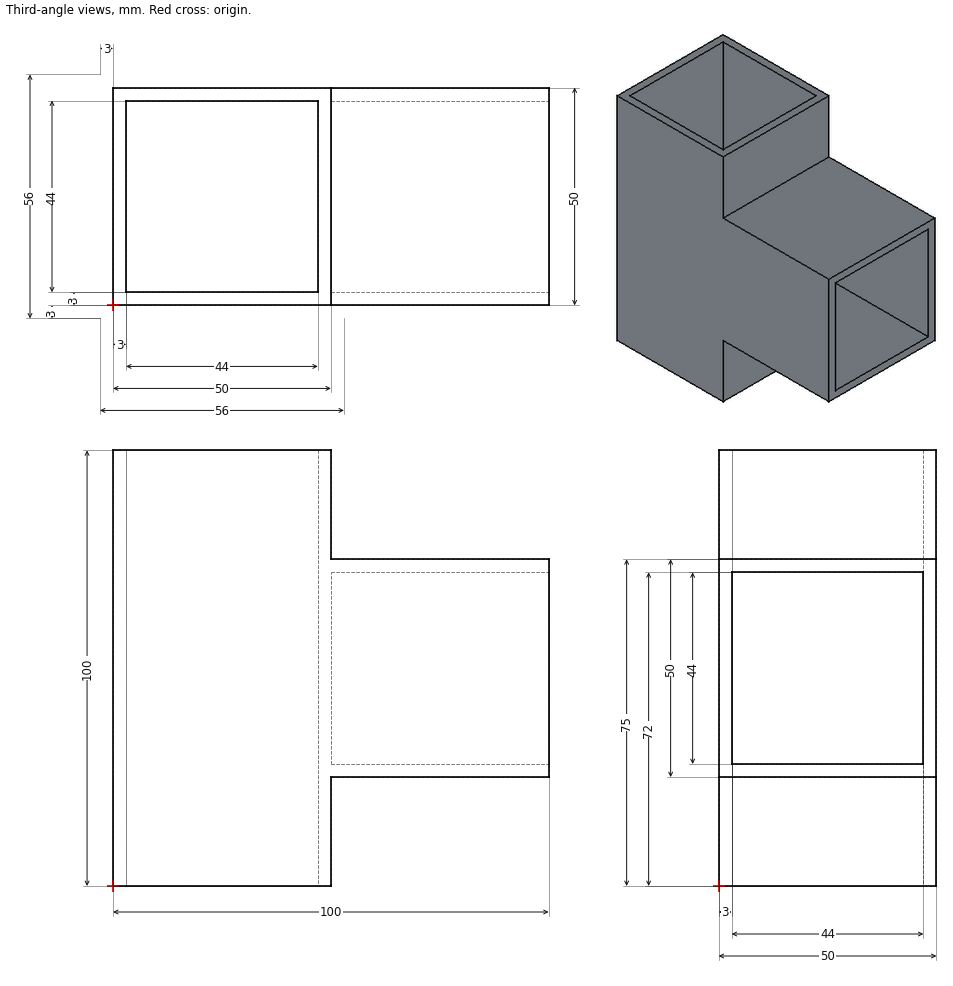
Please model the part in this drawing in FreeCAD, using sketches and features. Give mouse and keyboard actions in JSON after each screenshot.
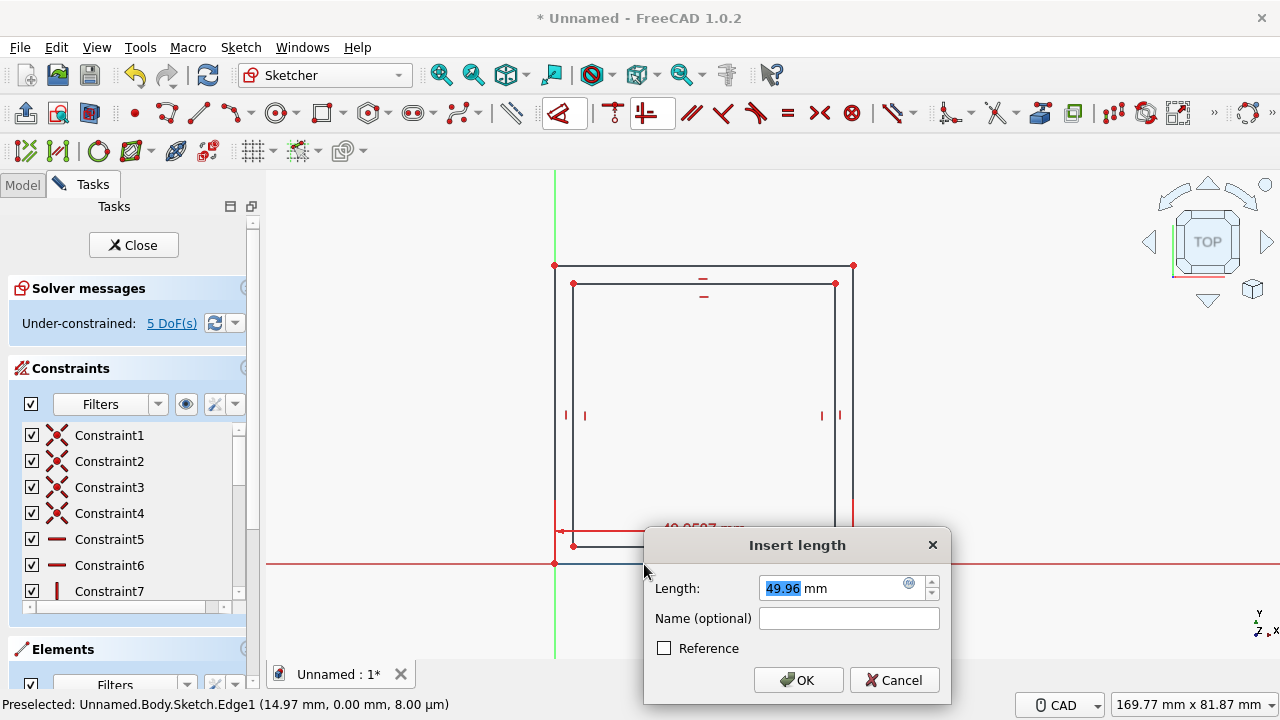
{"action": "type", "text": "50"}
{"action": "key", "text": "Return"}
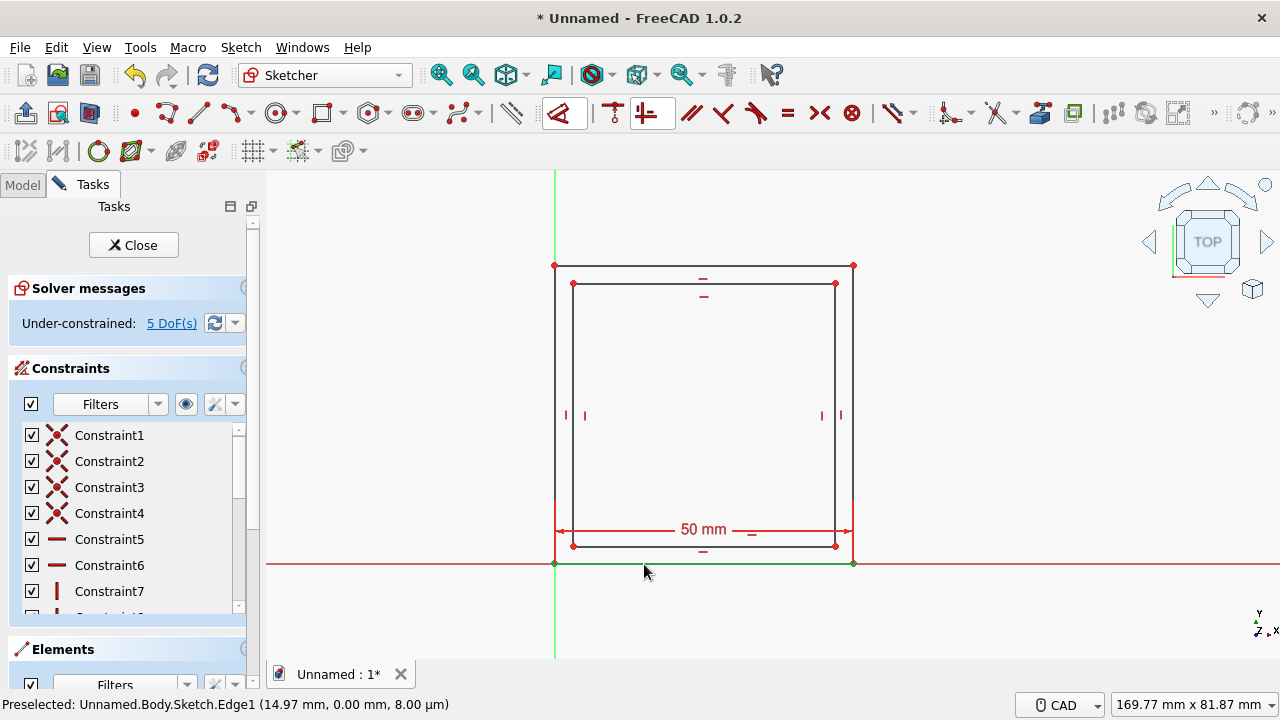
{"action": "left_click", "coordinate": [853, 475]}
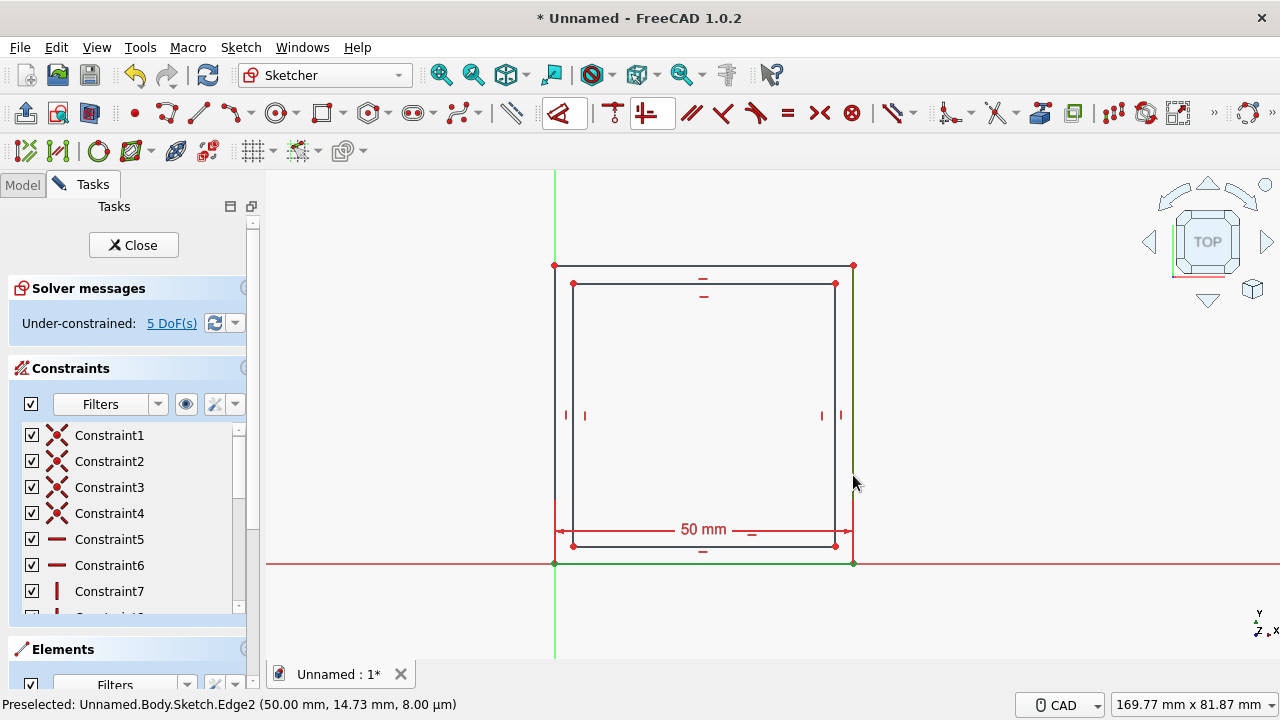
{"action": "key", "text": "i"}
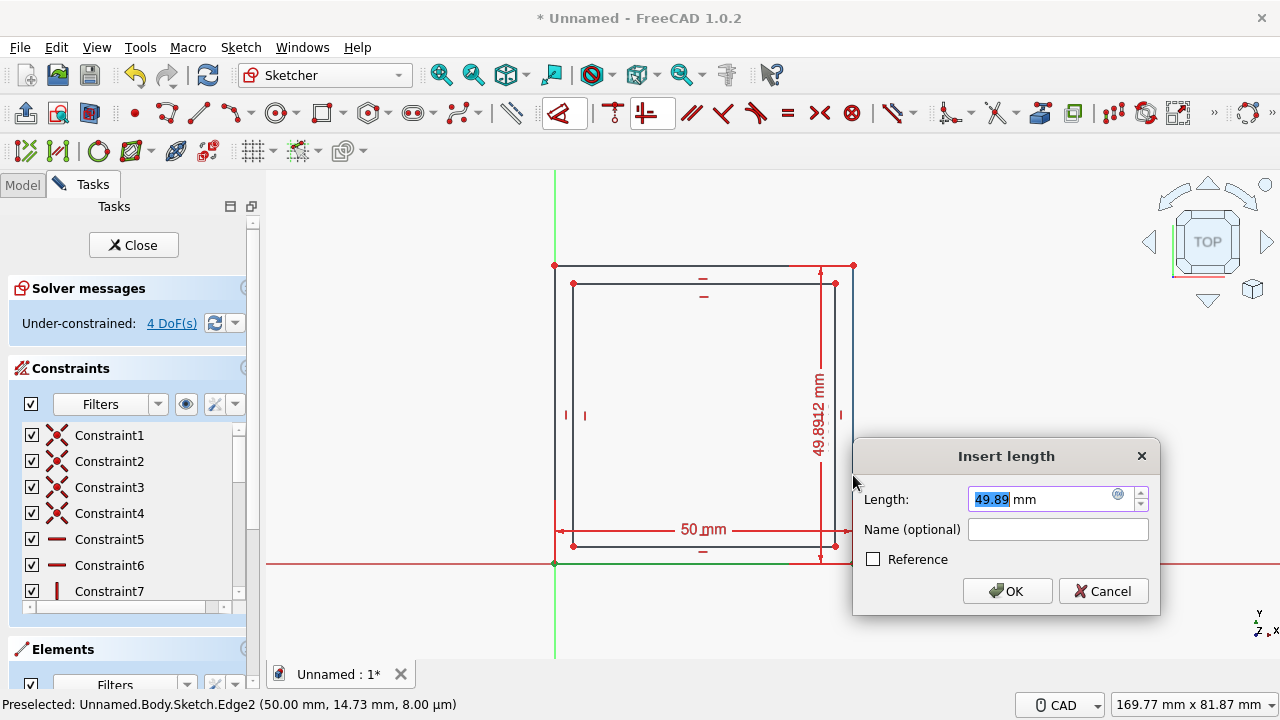
{"action": "type", "text": "50"}
{"action": "key", "text": "Return"}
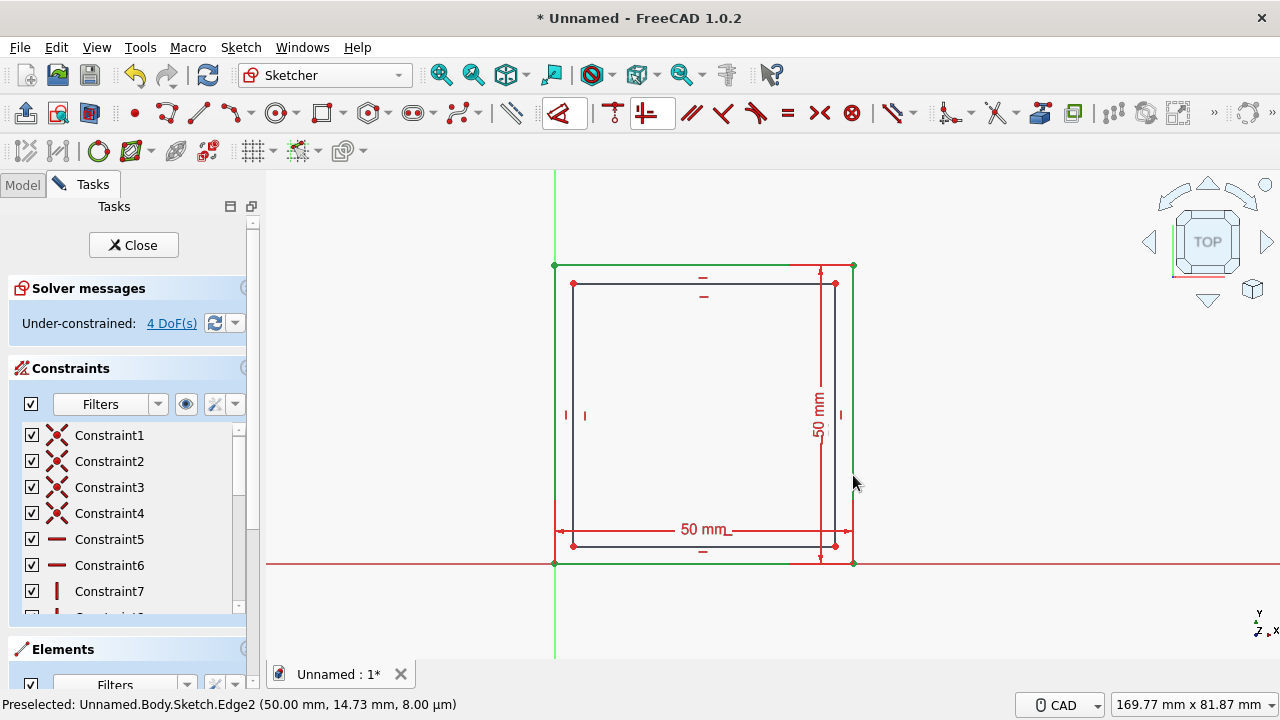
{"action": "left_click", "coordinate": [573, 363]}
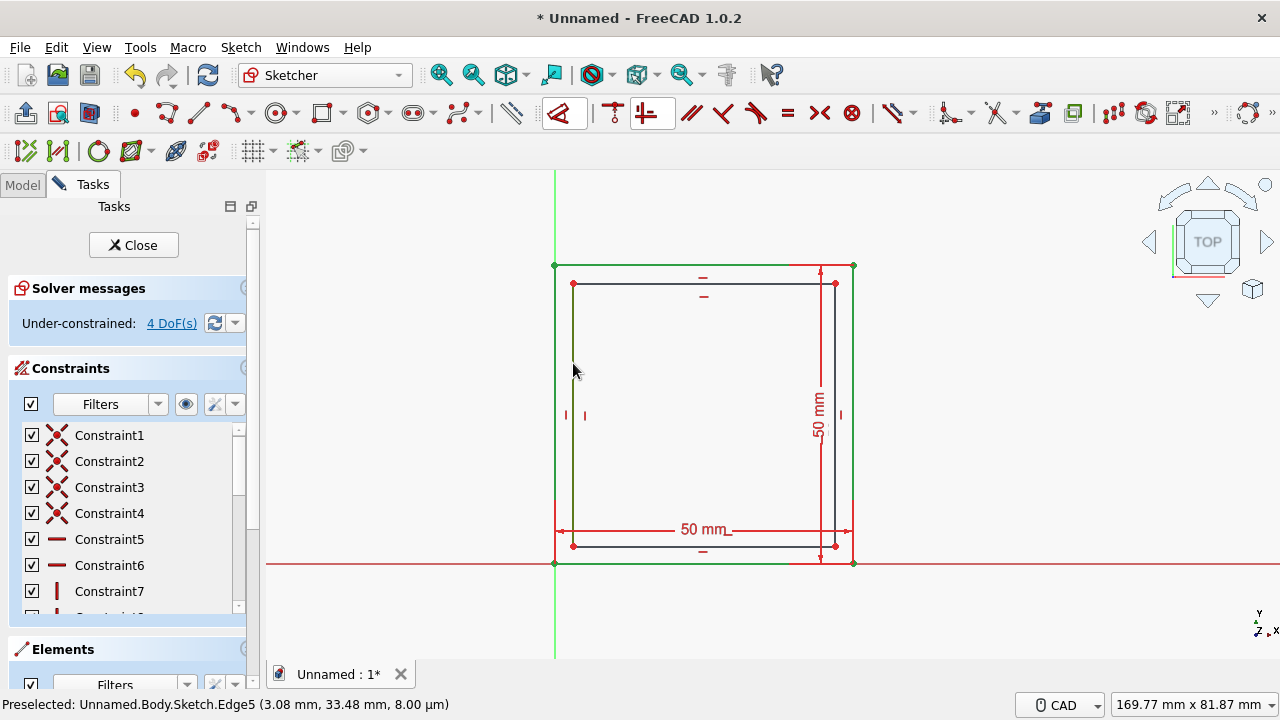
{"action": "key", "text": "i"}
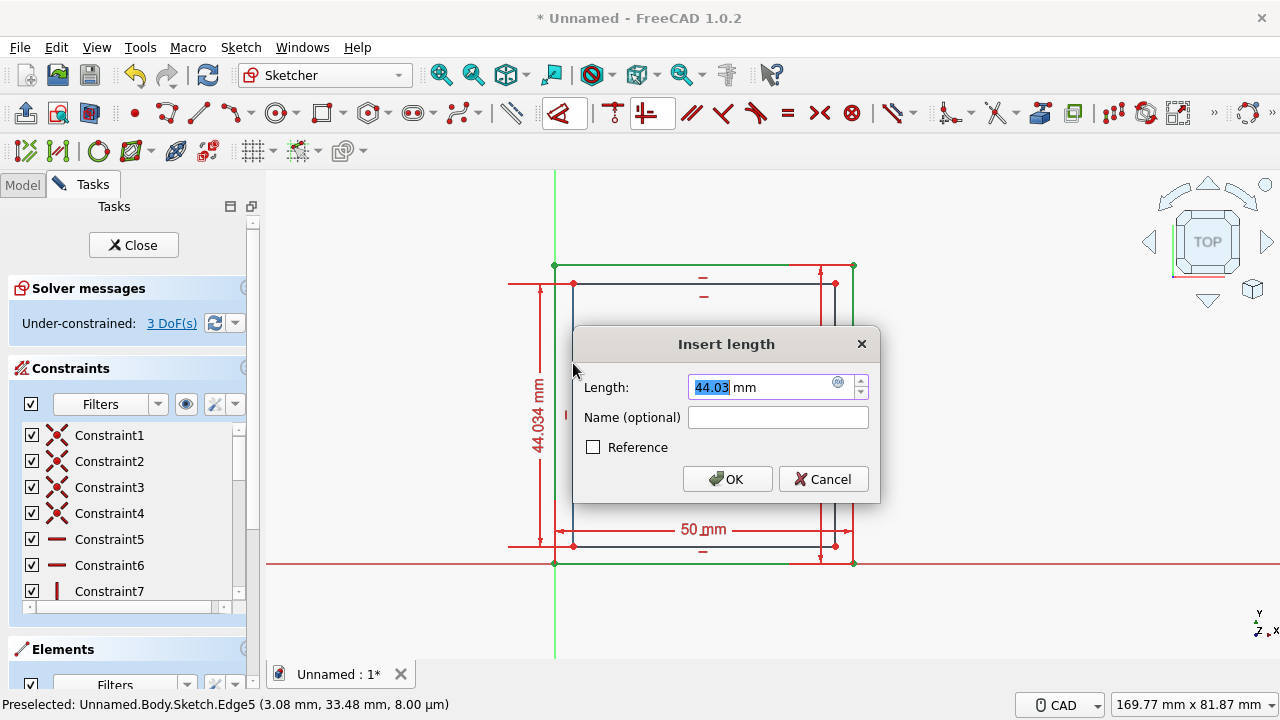
{"action": "type", "text": "44"}
{"action": "key", "text": "Return"}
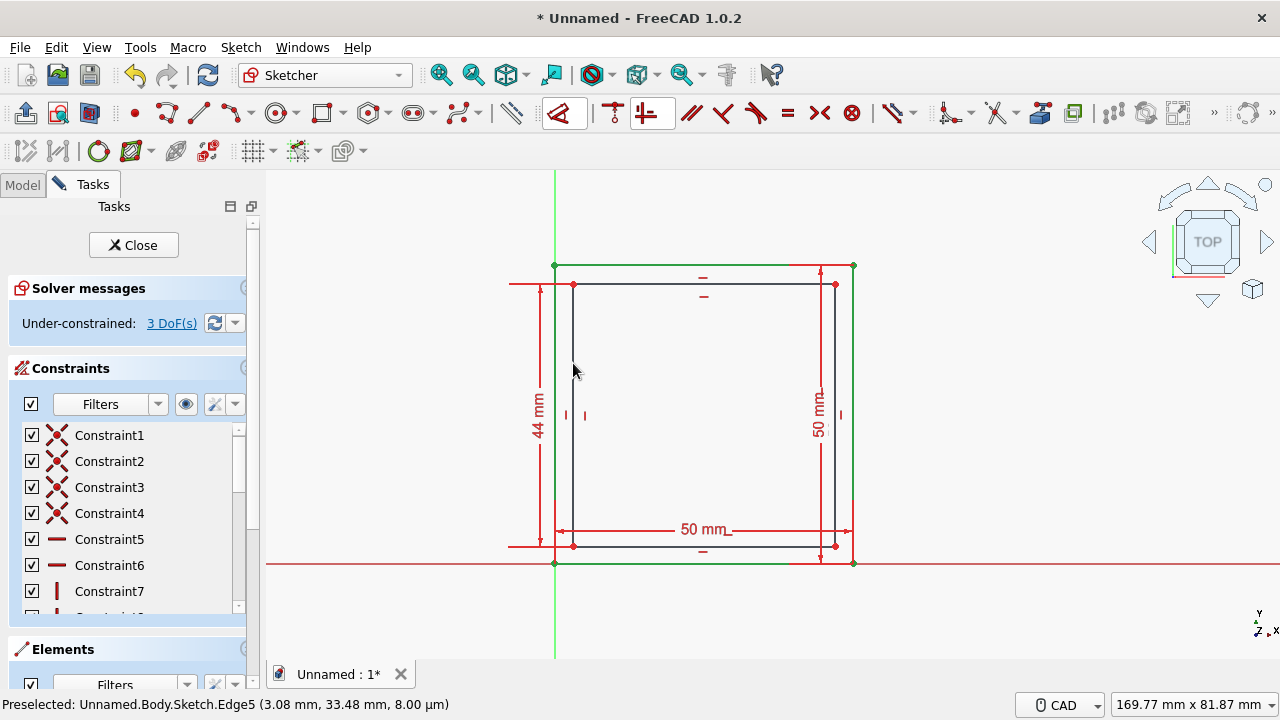
{"action": "left_click", "coordinate": [652, 547]}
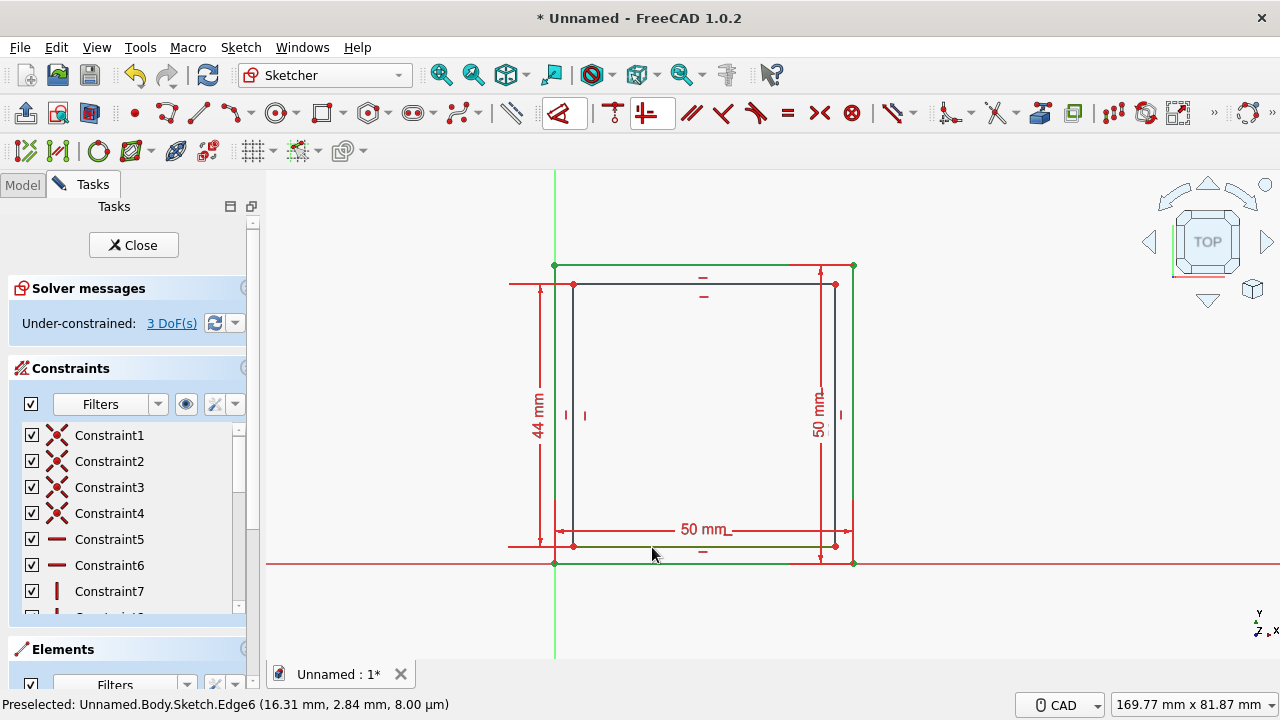
{"action": "key", "text": "l"}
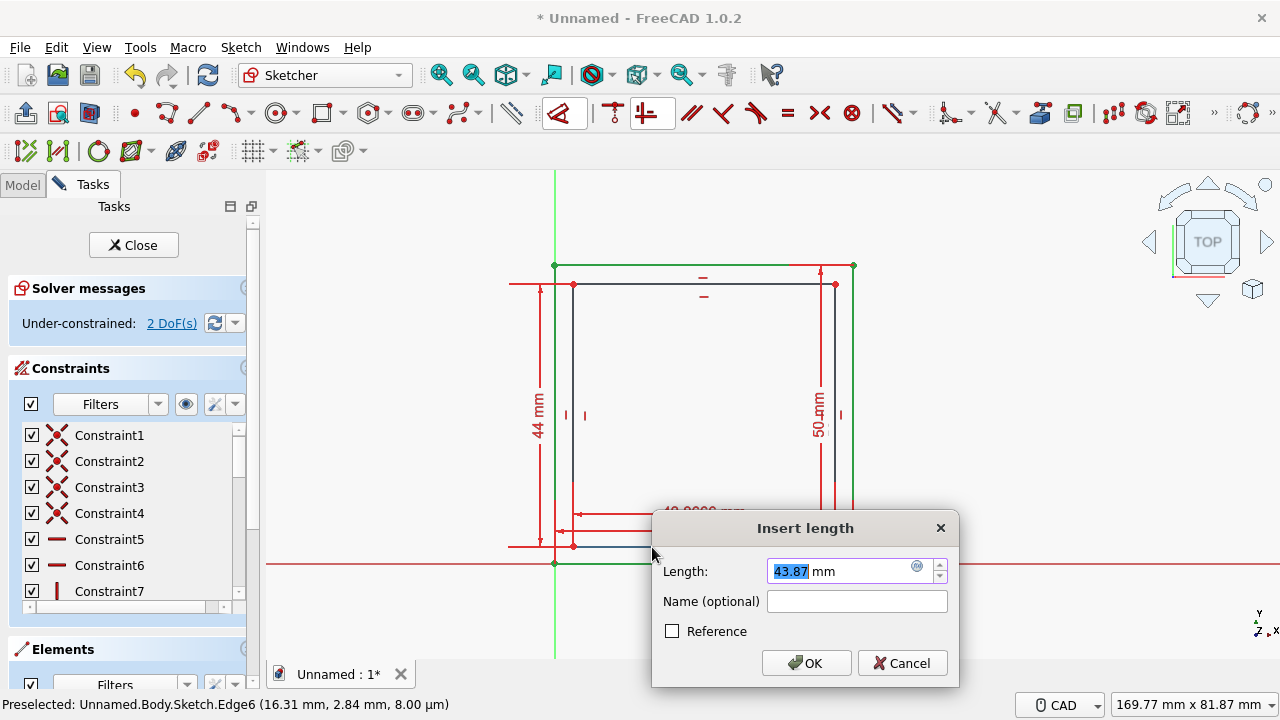
{"action": "type", "text": "44"}
{"action": "key", "text": "Return"}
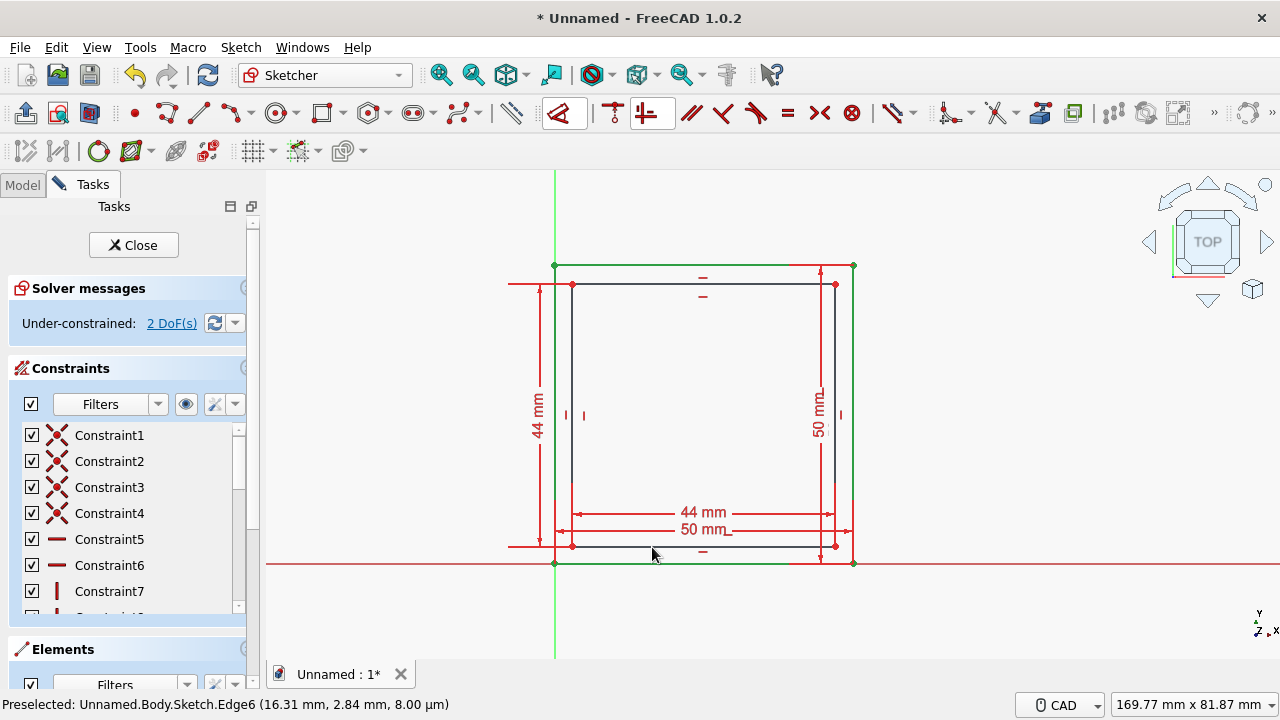
{"action": "scroll", "coordinate": [572, 284], "scroll_direction": "up", "scroll_amount": 4}